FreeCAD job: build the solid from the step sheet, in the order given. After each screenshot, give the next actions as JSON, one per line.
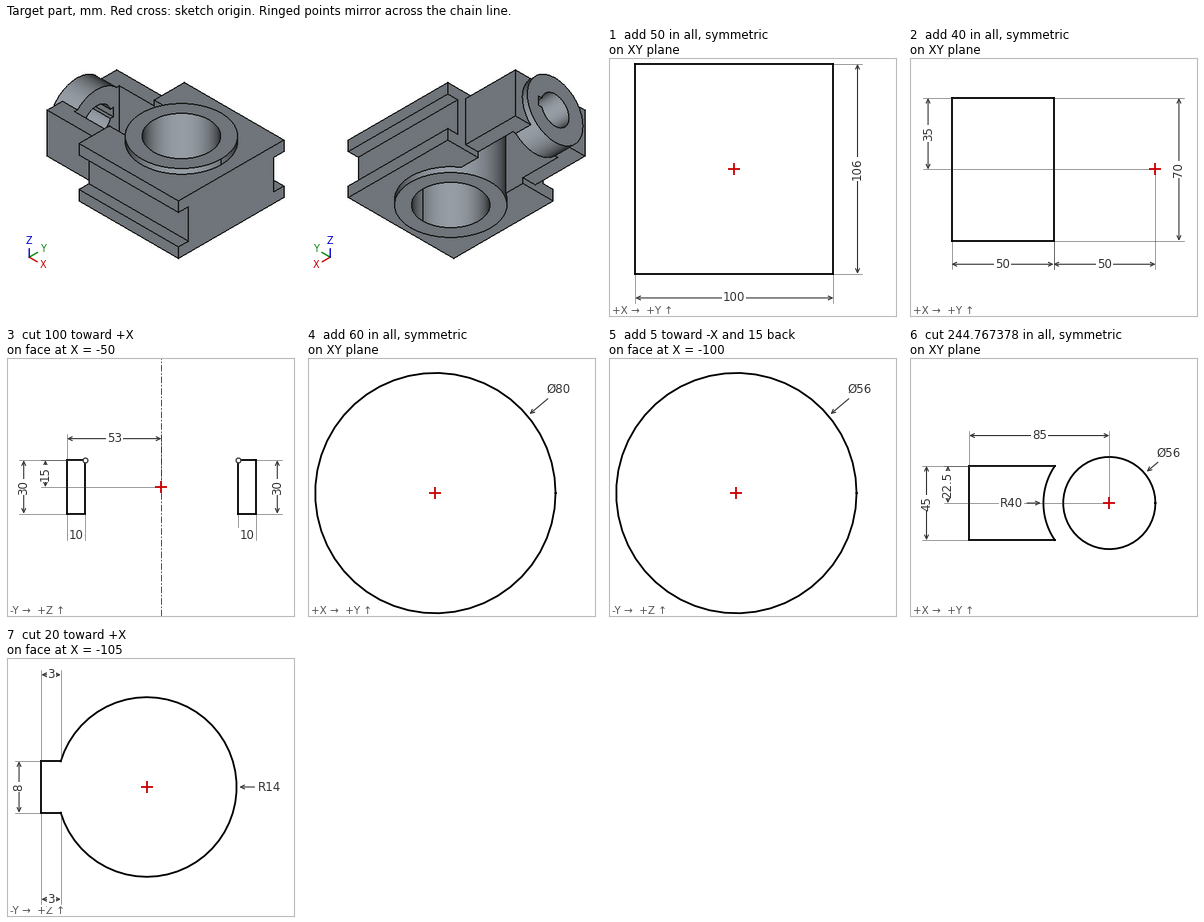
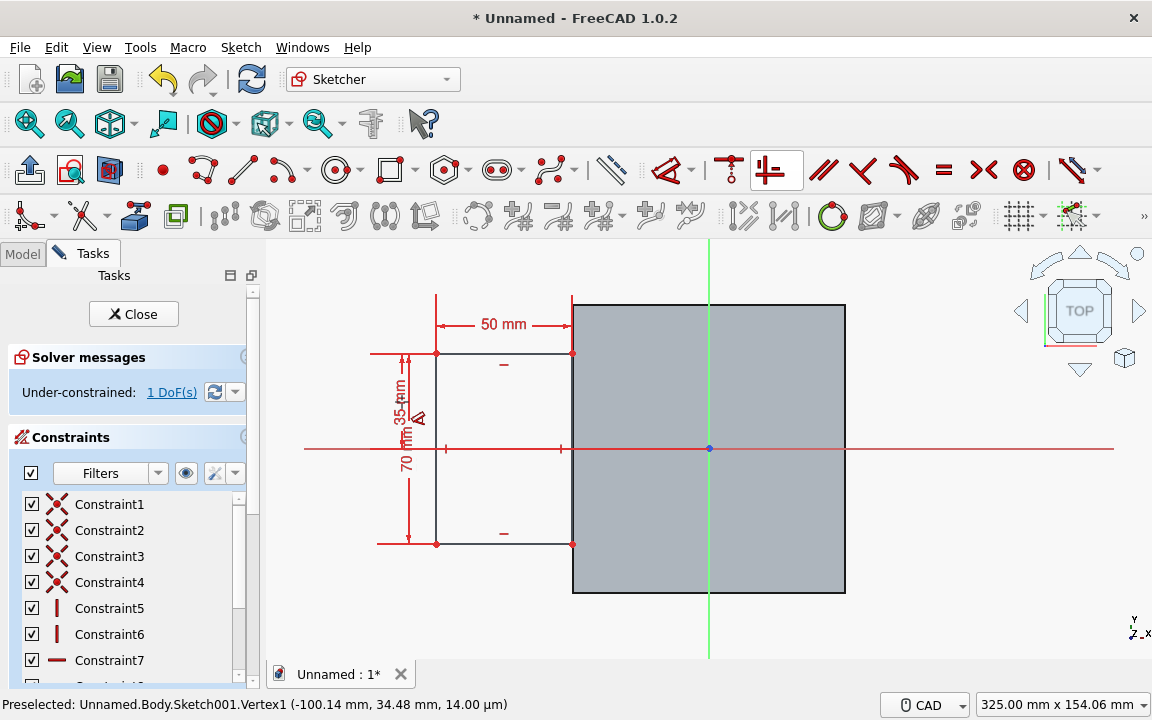
{"action": "left_click", "coordinate": [572, 544]}
{"action": "left_click", "coordinate": [641, 578]}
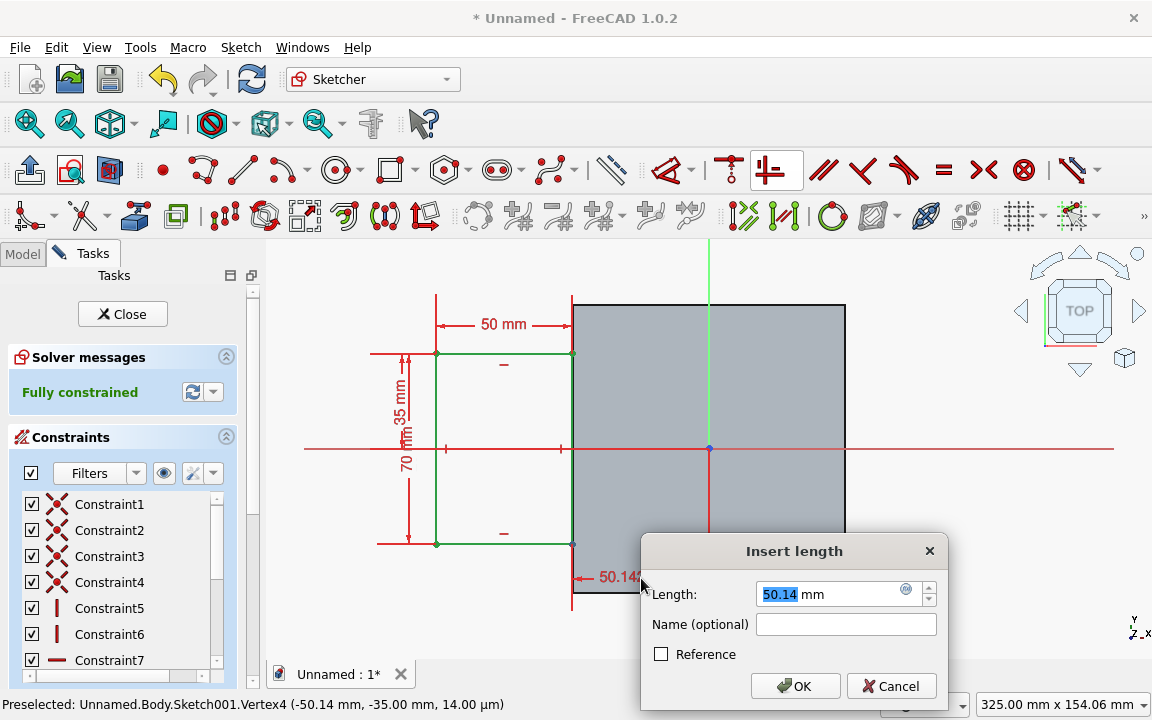
{"action": "type", "text": "50"}
{"action": "key", "text": "Return"}
{"action": "key", "text": "Escape"}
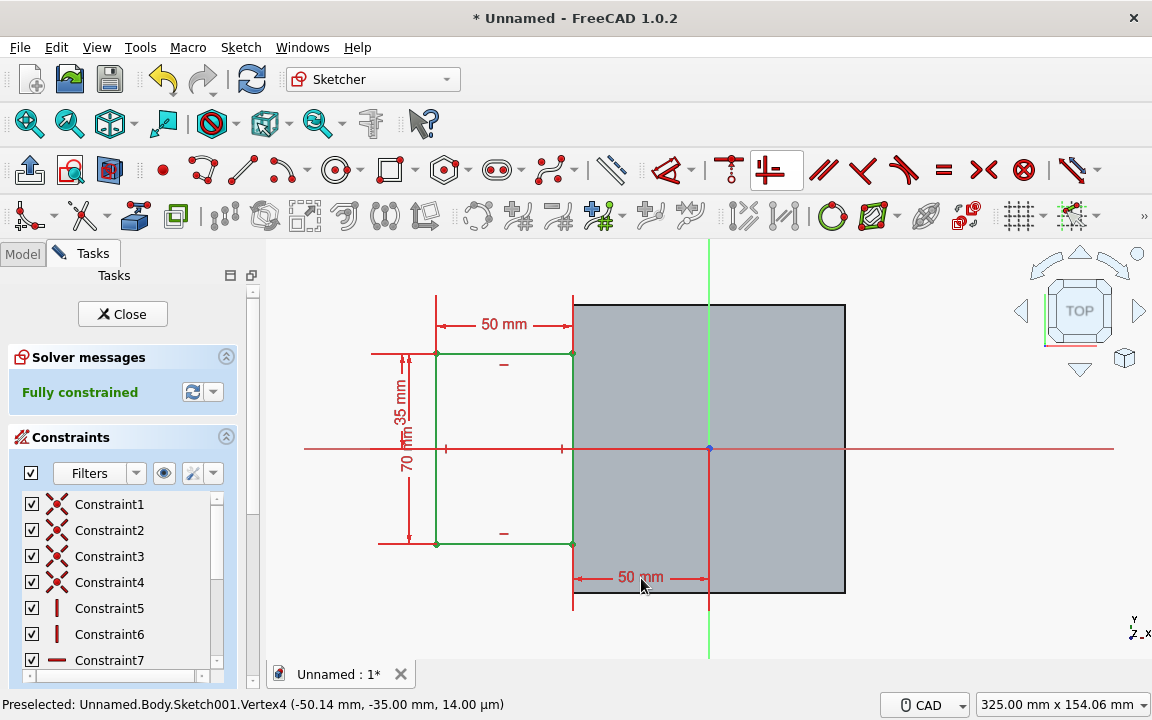
{"action": "left_click", "coordinate": [123, 314]}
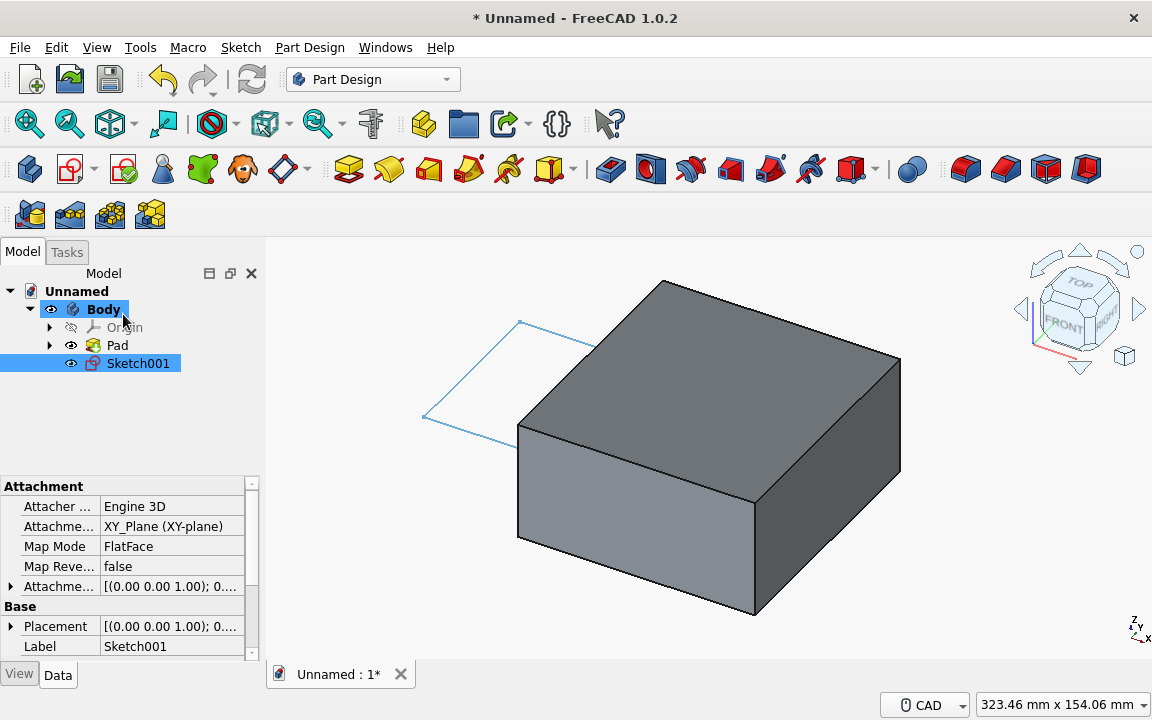
{"action": "left_click", "coordinate": [350, 170]}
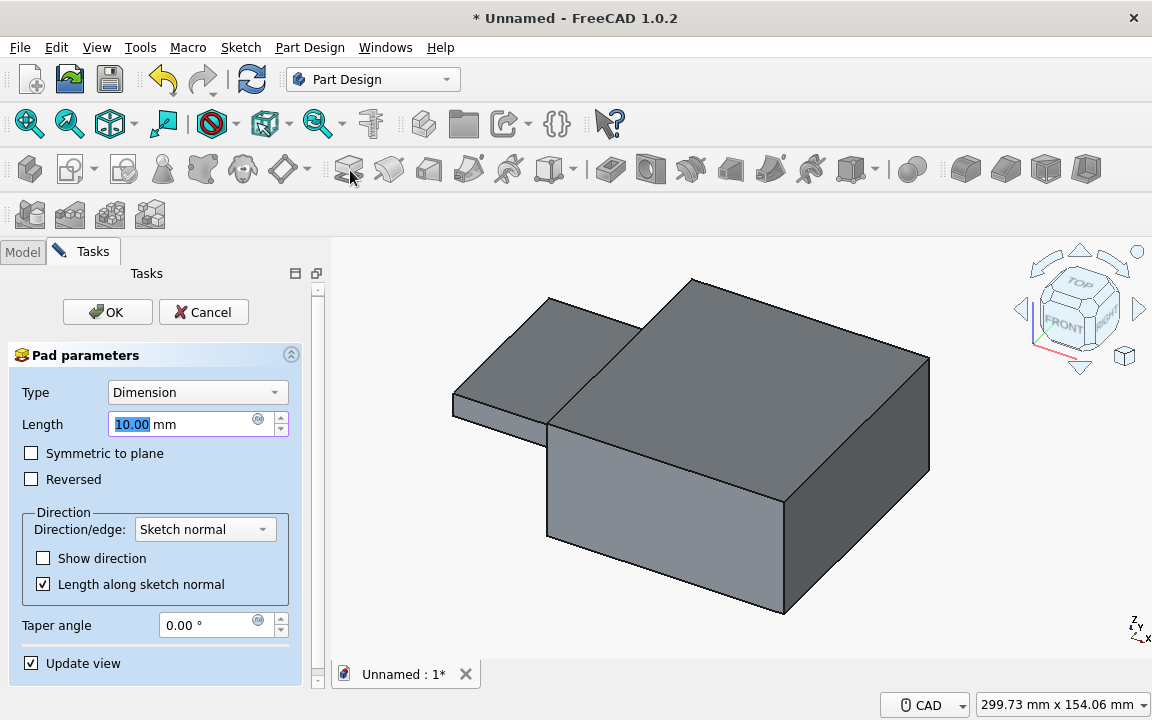
{"action": "type", "text": "40"}
{"action": "key", "text": "Tab"}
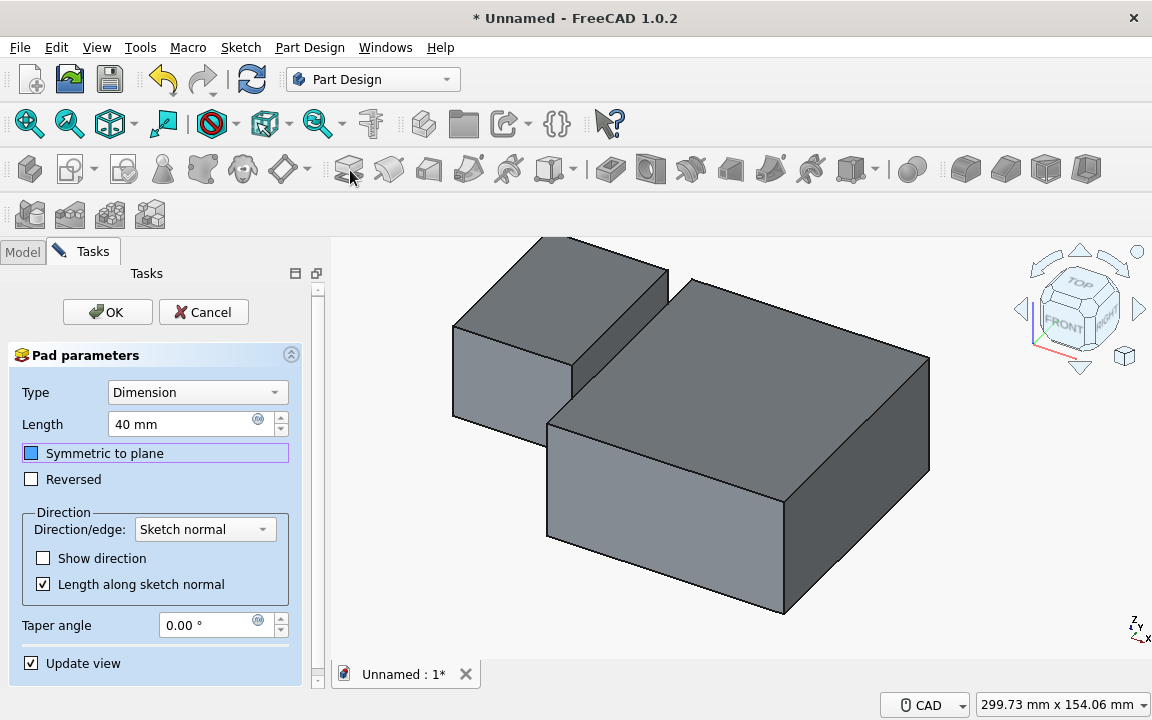
{"action": "left_click", "coordinate": [30, 453]}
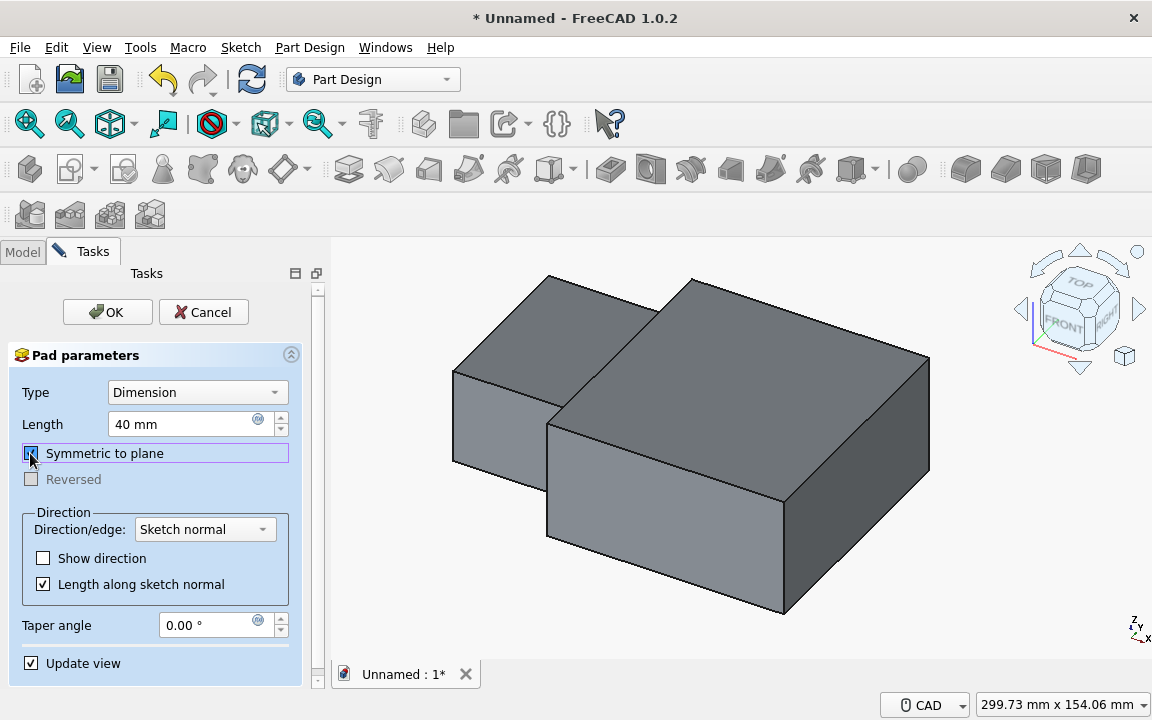
{"action": "left_click", "coordinate": [108, 312]}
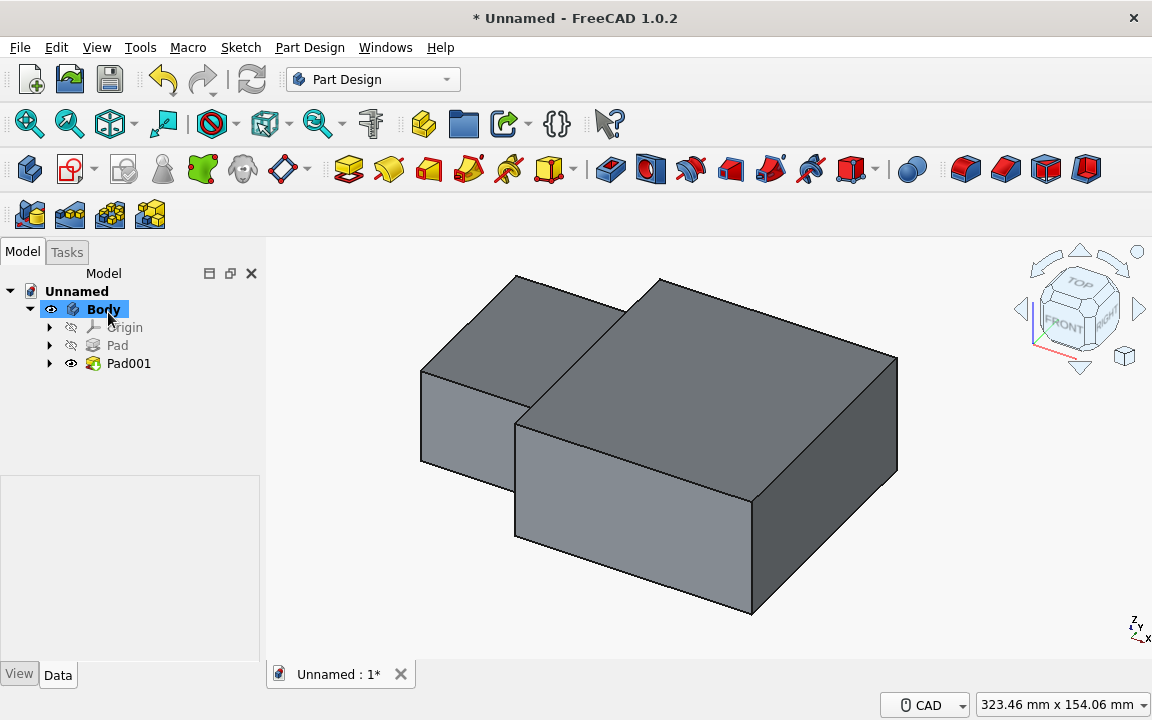
{"action": "key", "text": "6"}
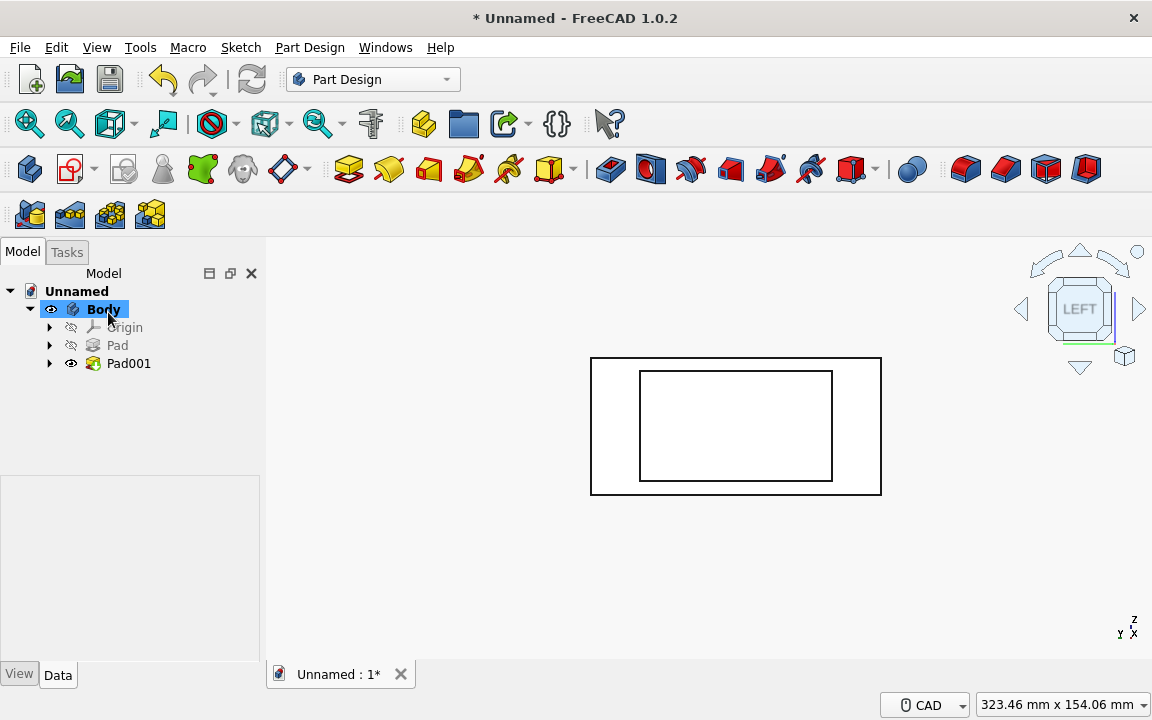
{"action": "left_click", "coordinate": [30, 124]}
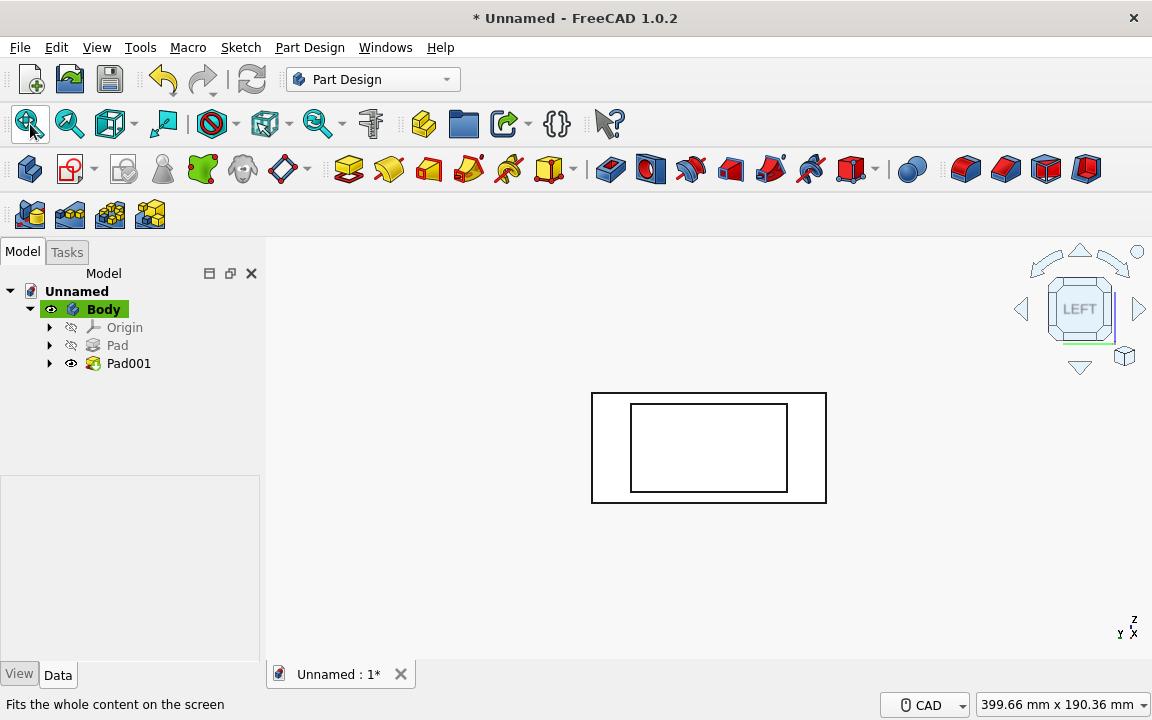
{"action": "left_click", "coordinate": [608, 415]}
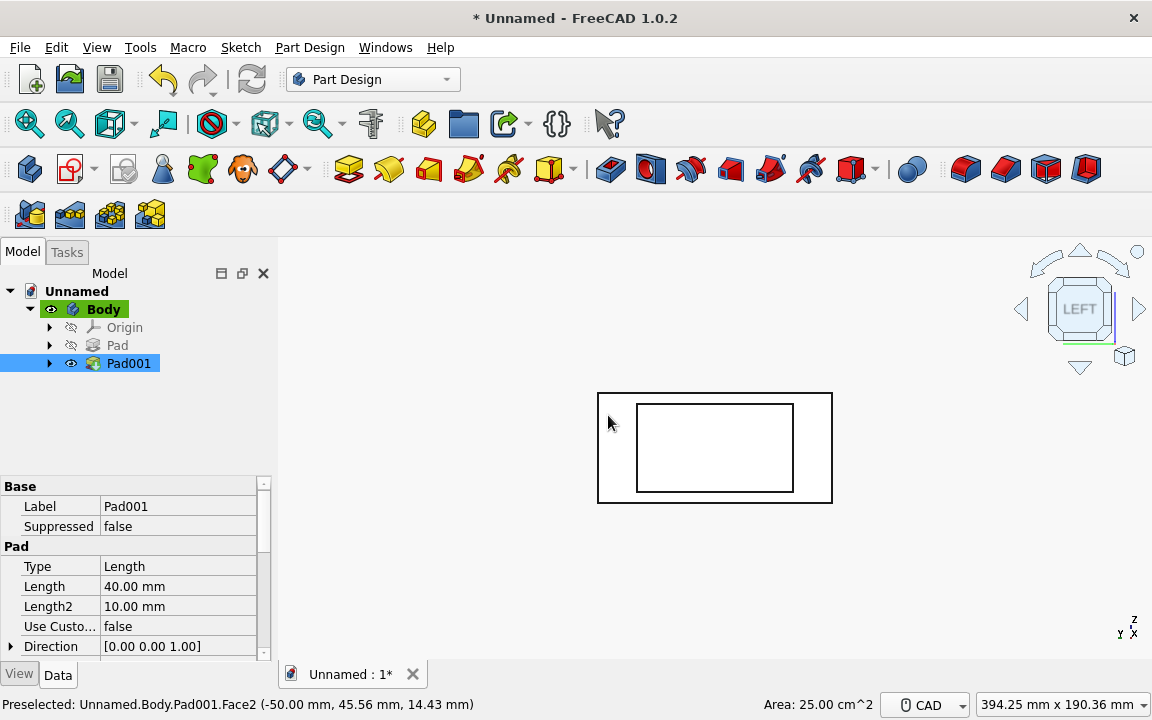
{"action": "left_click", "coordinate": [70, 170]}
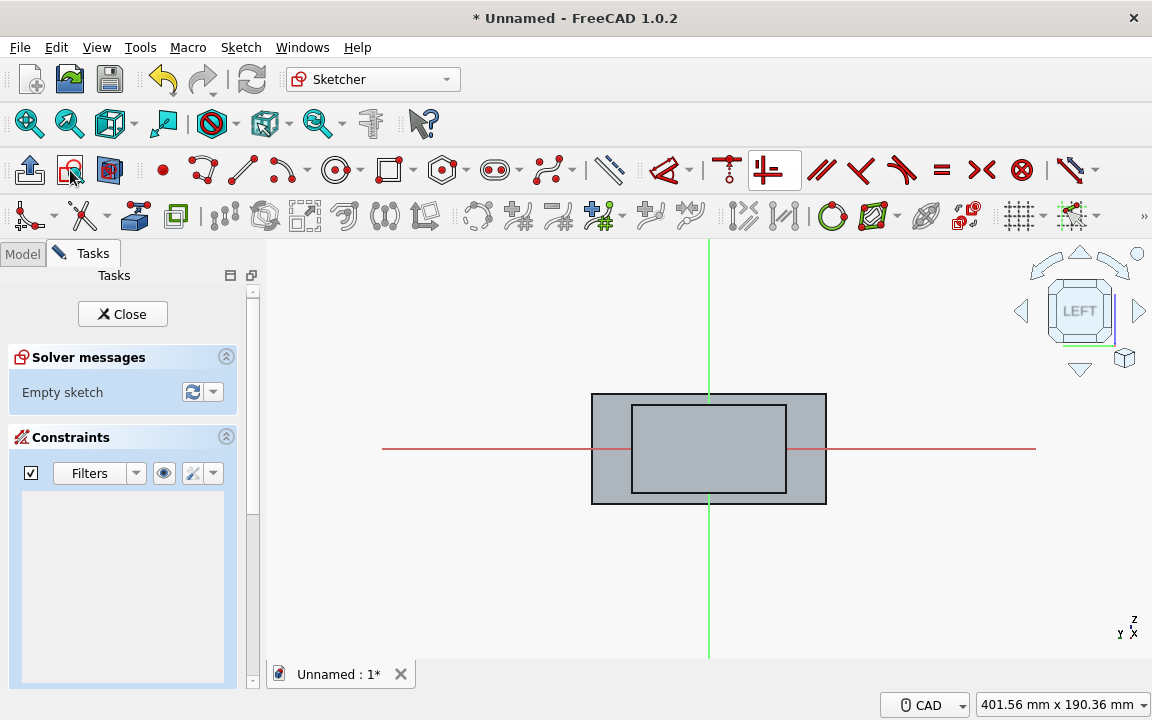
{"action": "scroll", "coordinate": [765, 449], "scroll_direction": "up", "scroll_amount": 4}